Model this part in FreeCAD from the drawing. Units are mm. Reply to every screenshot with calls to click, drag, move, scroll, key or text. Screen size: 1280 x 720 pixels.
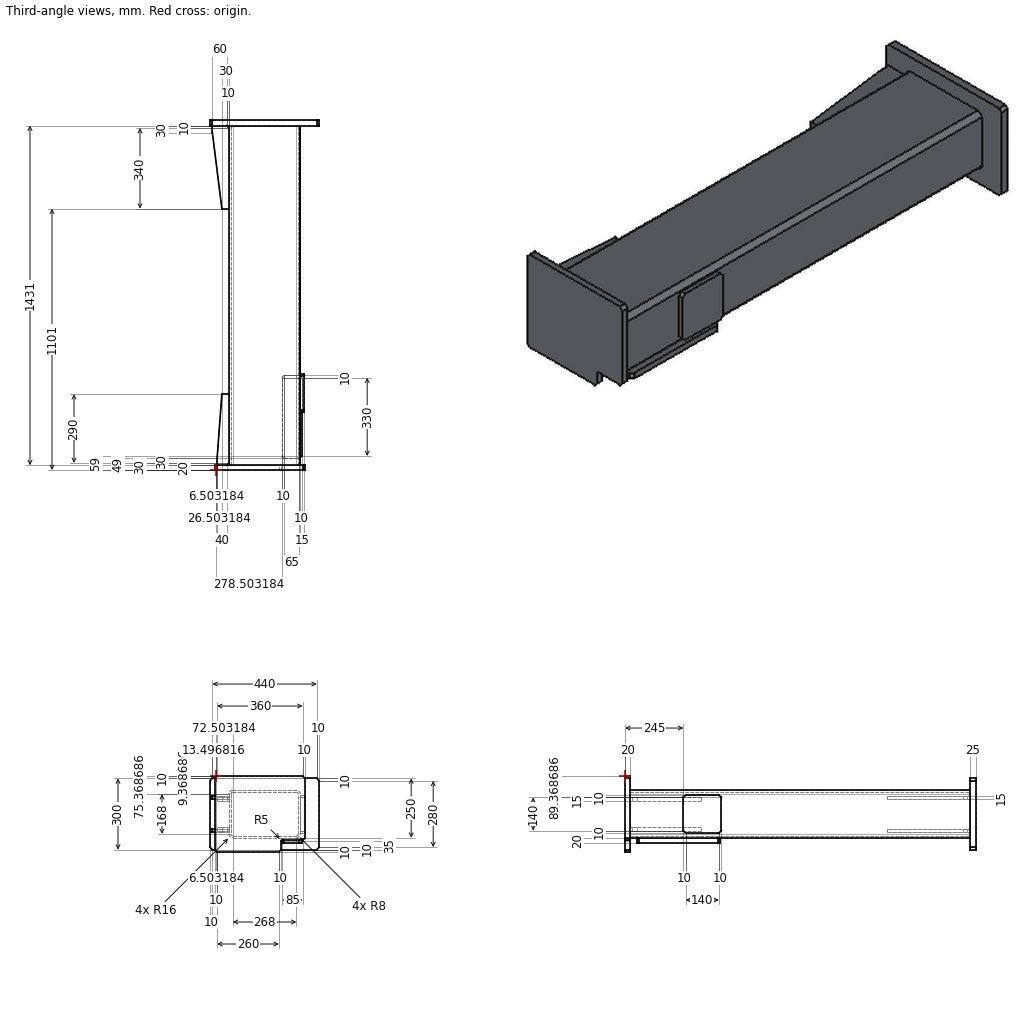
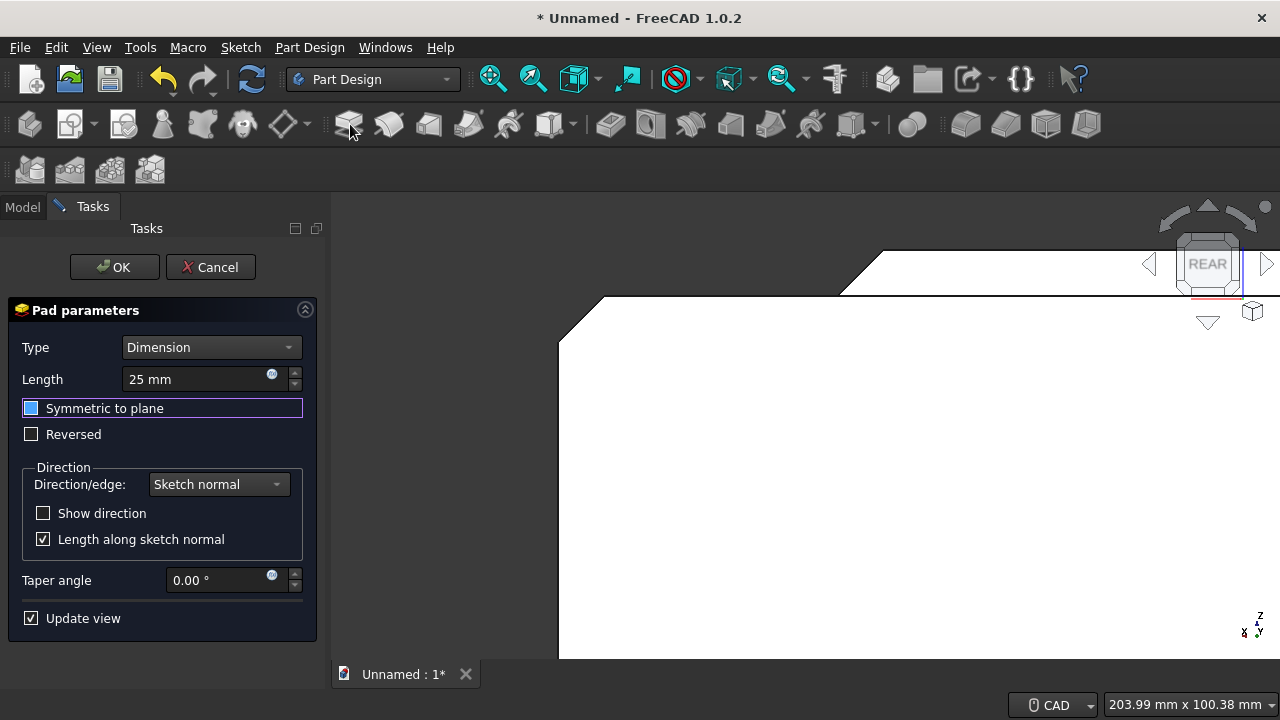
click(115, 267)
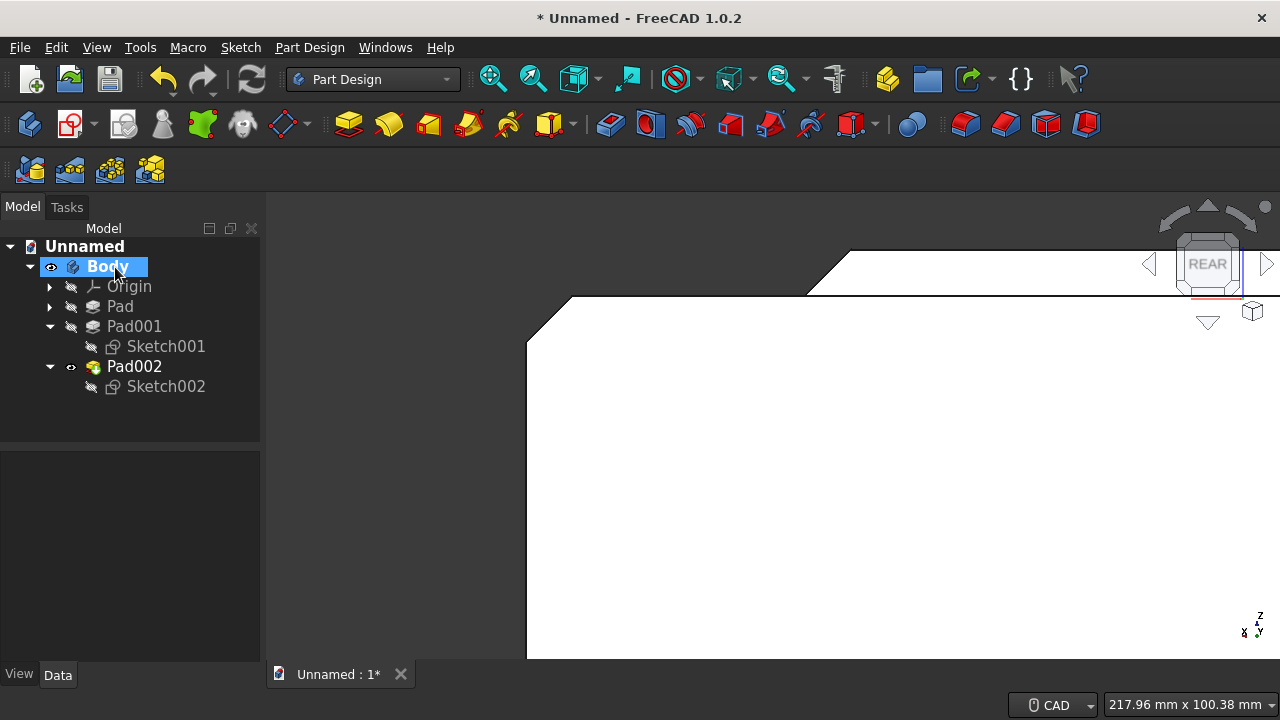
click(494, 80)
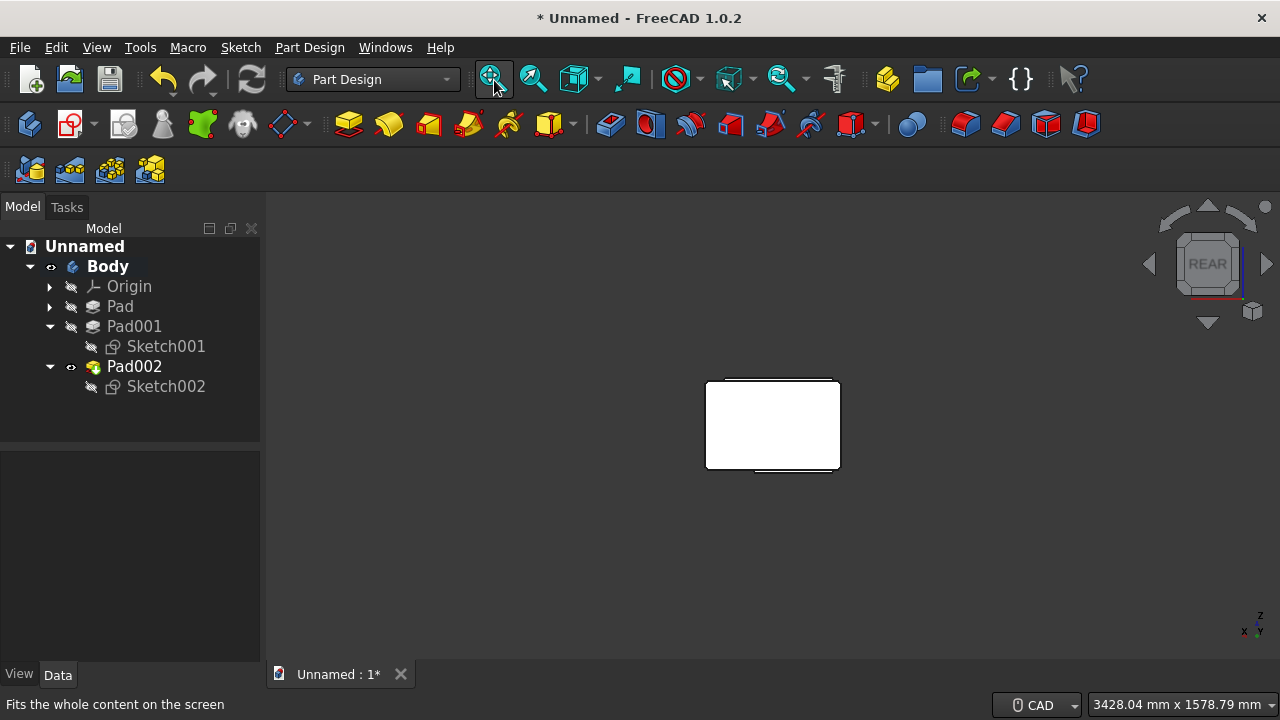
click(50, 287)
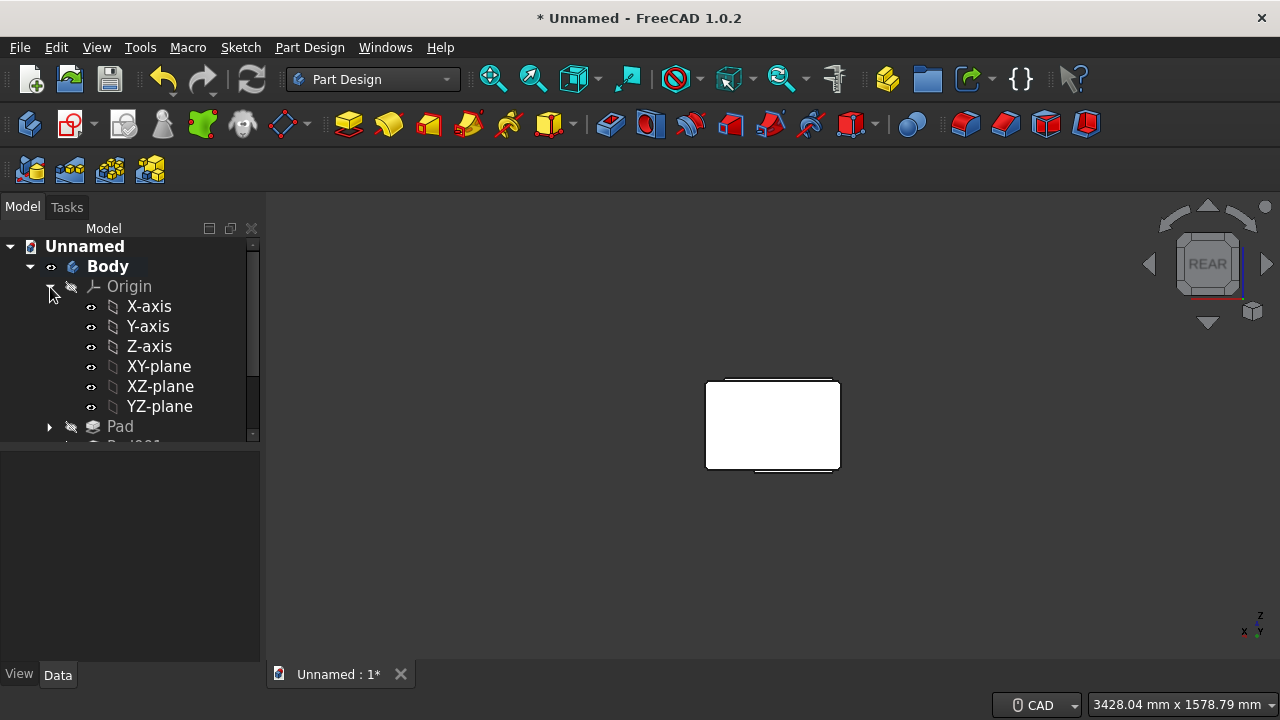
click(136, 367)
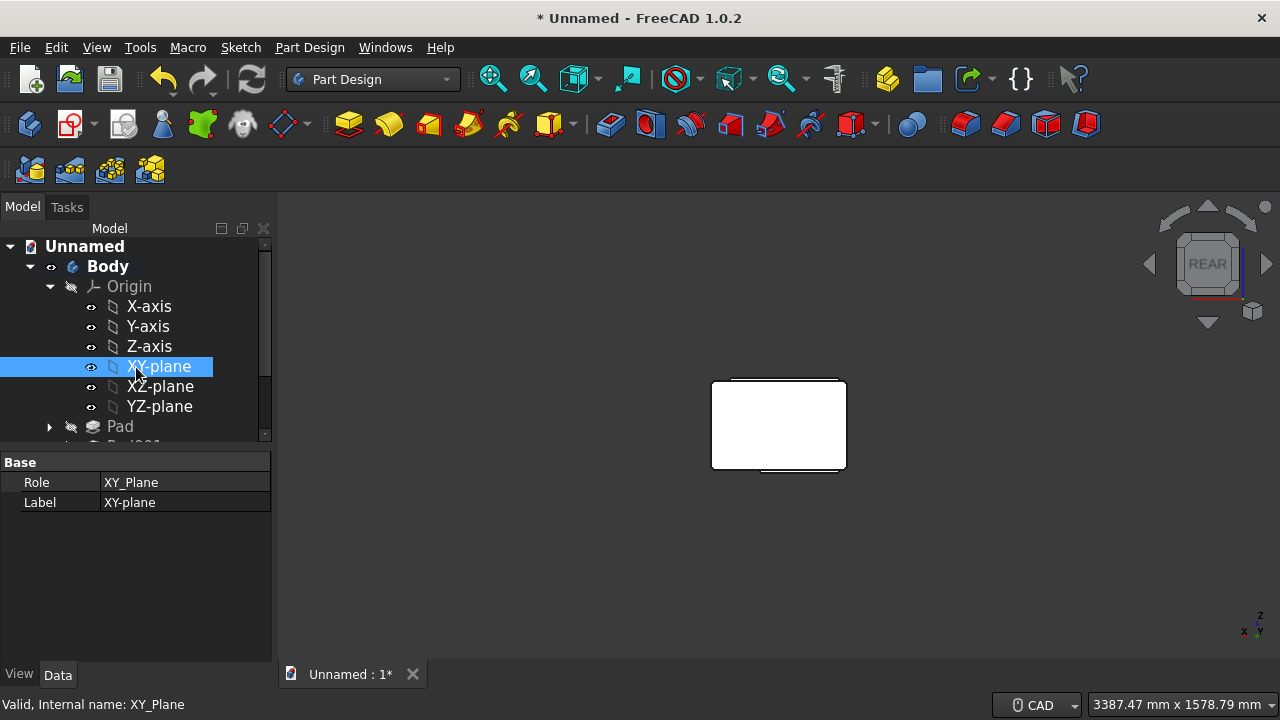
click(284, 124)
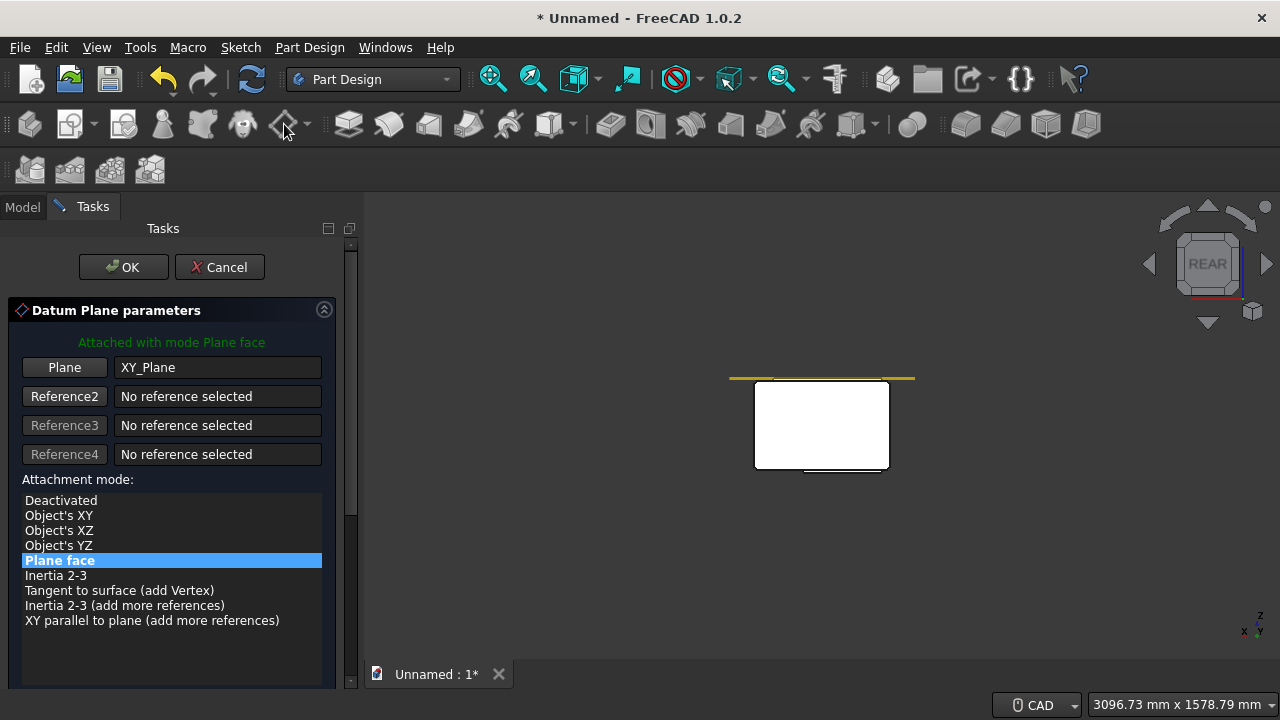
scroll(351, 463, down, 3)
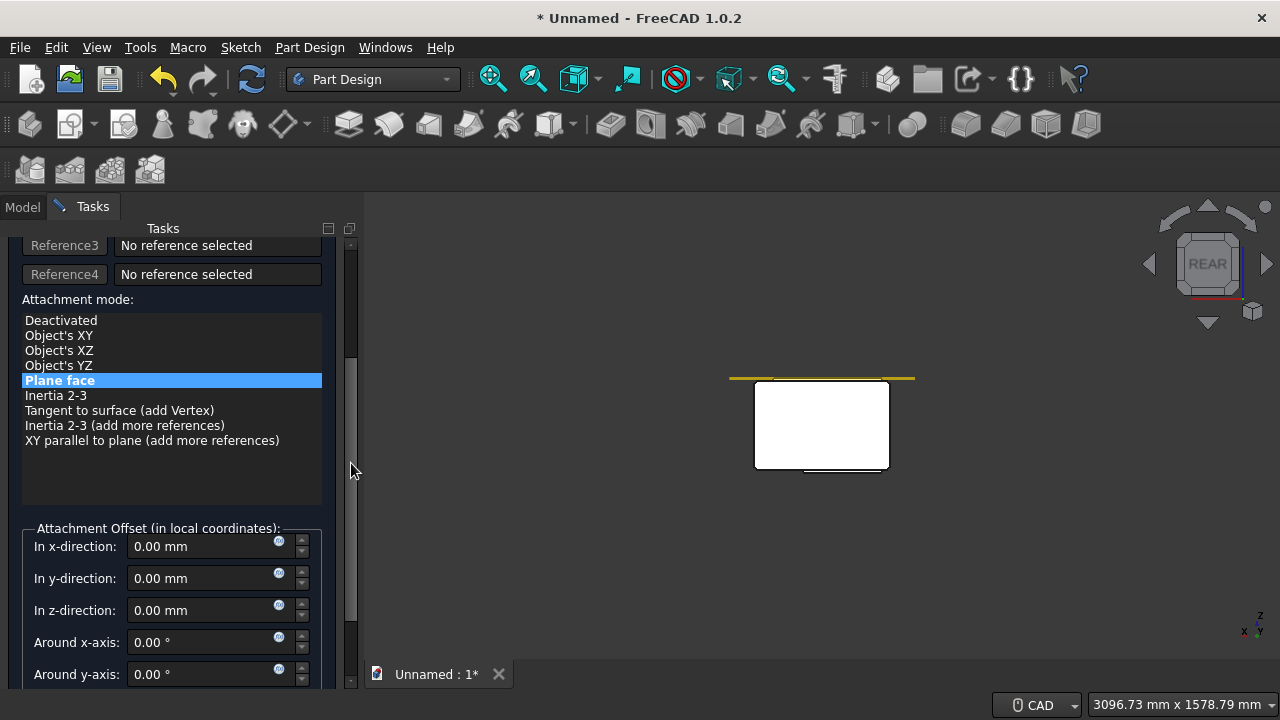
triple_click(210, 610)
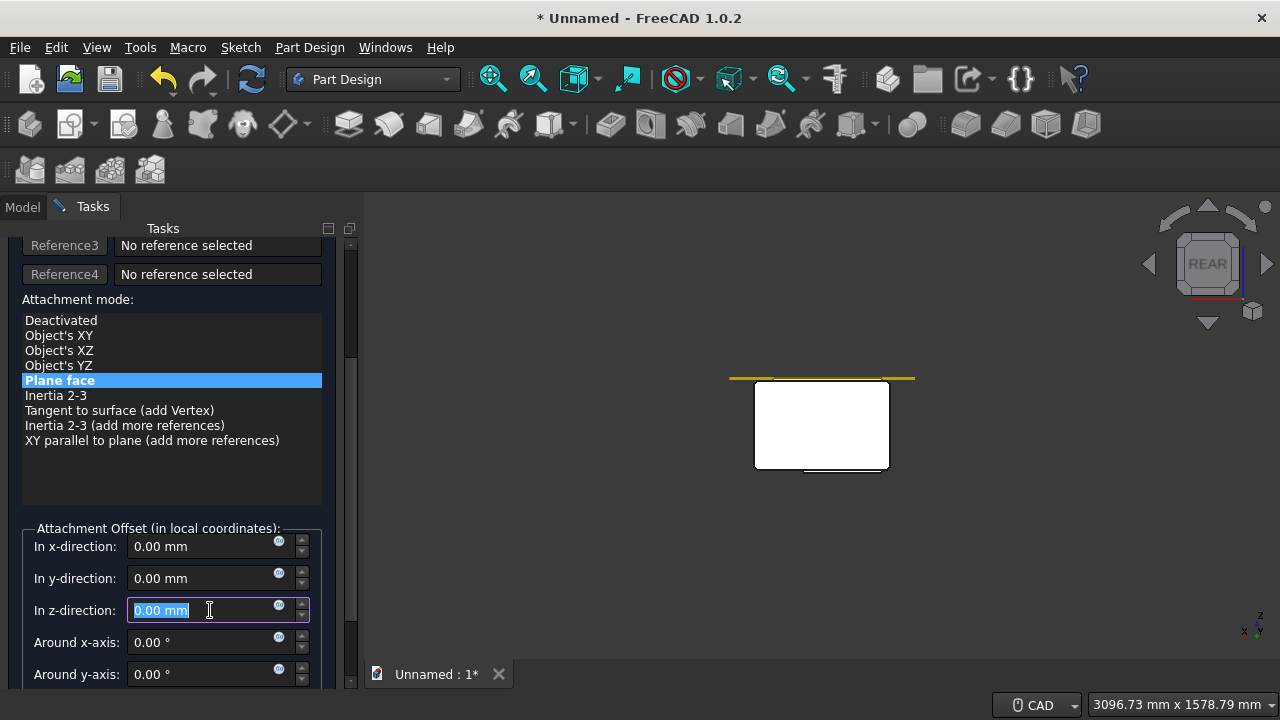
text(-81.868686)
key(Tab)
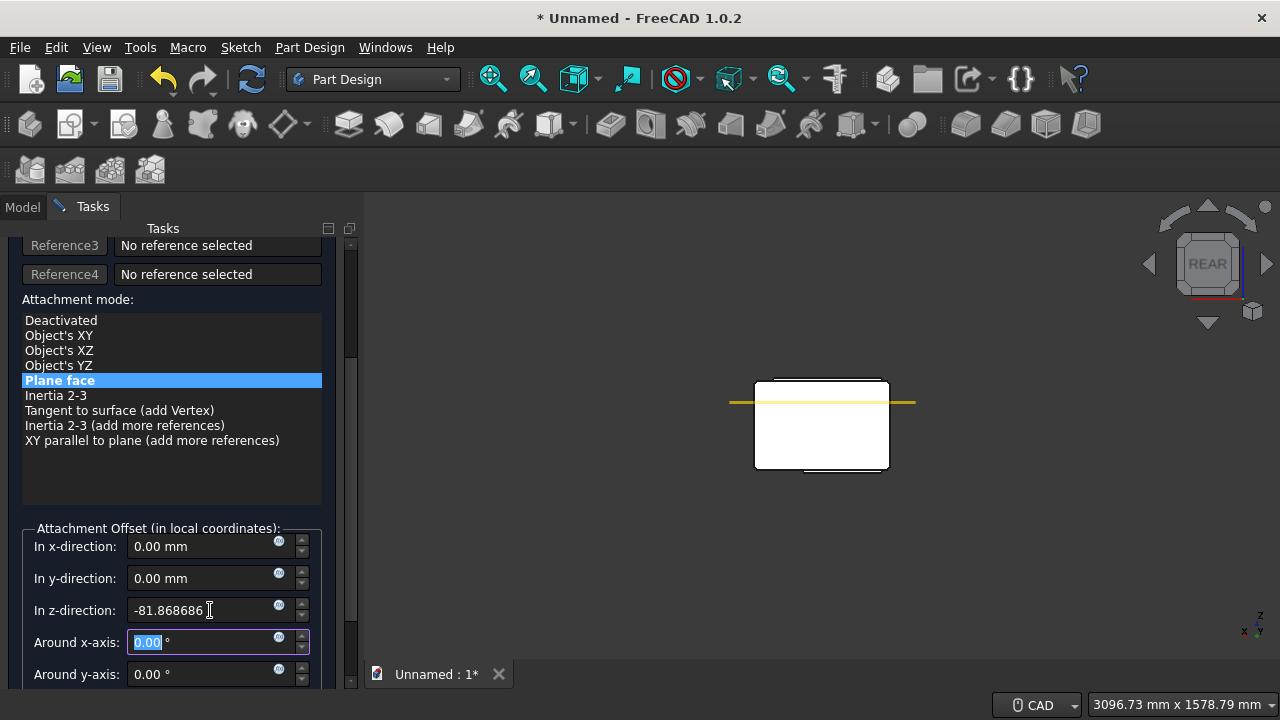
scroll(351, 463, up, 4)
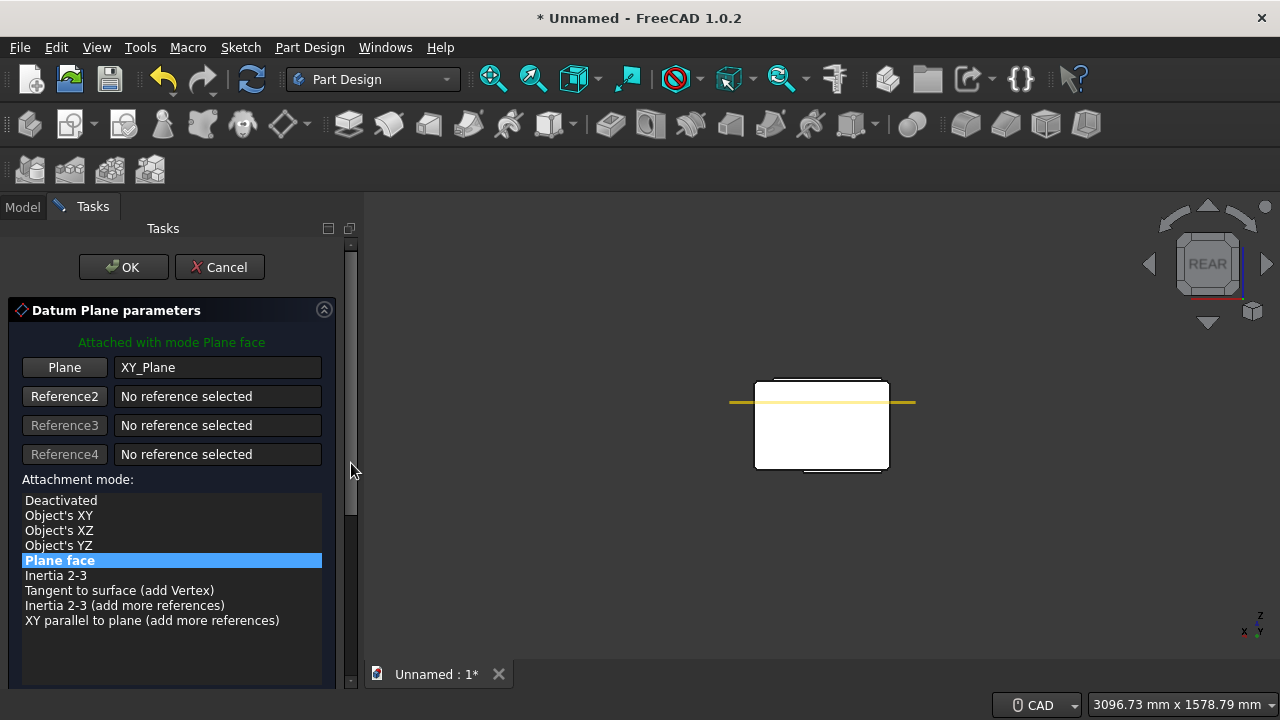
click(124, 267)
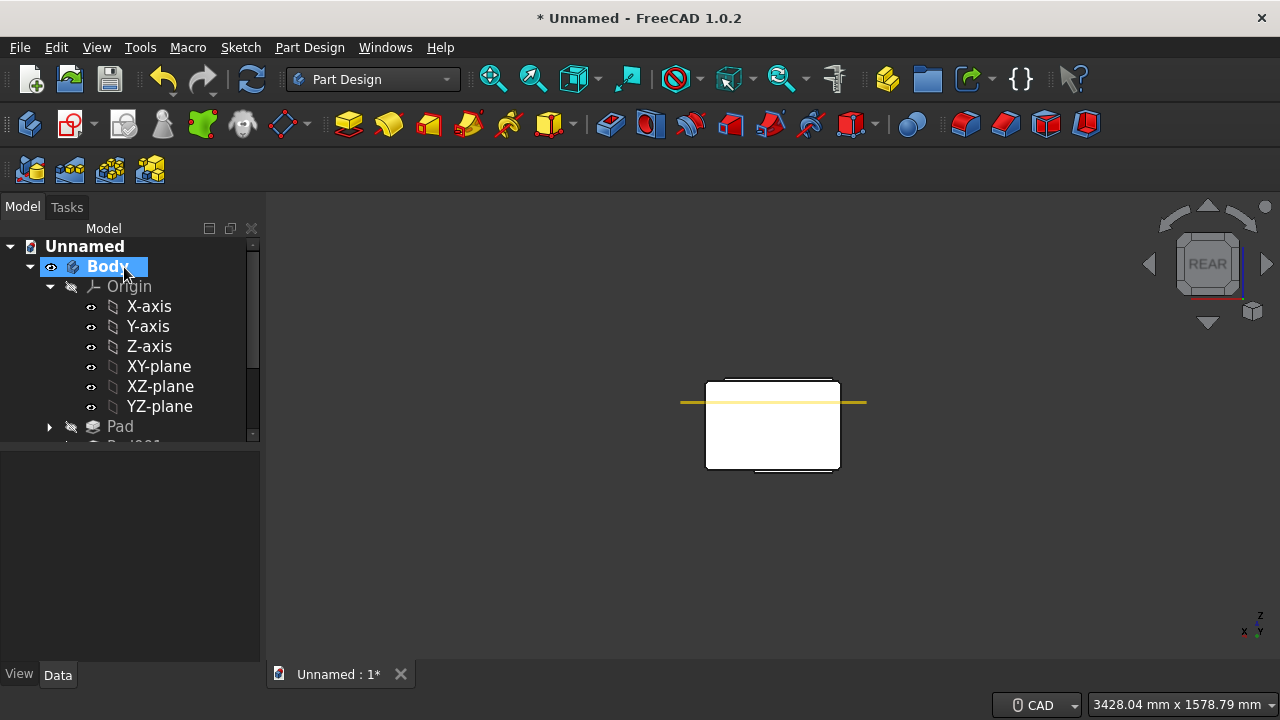
scroll(100, 342, down, 3)